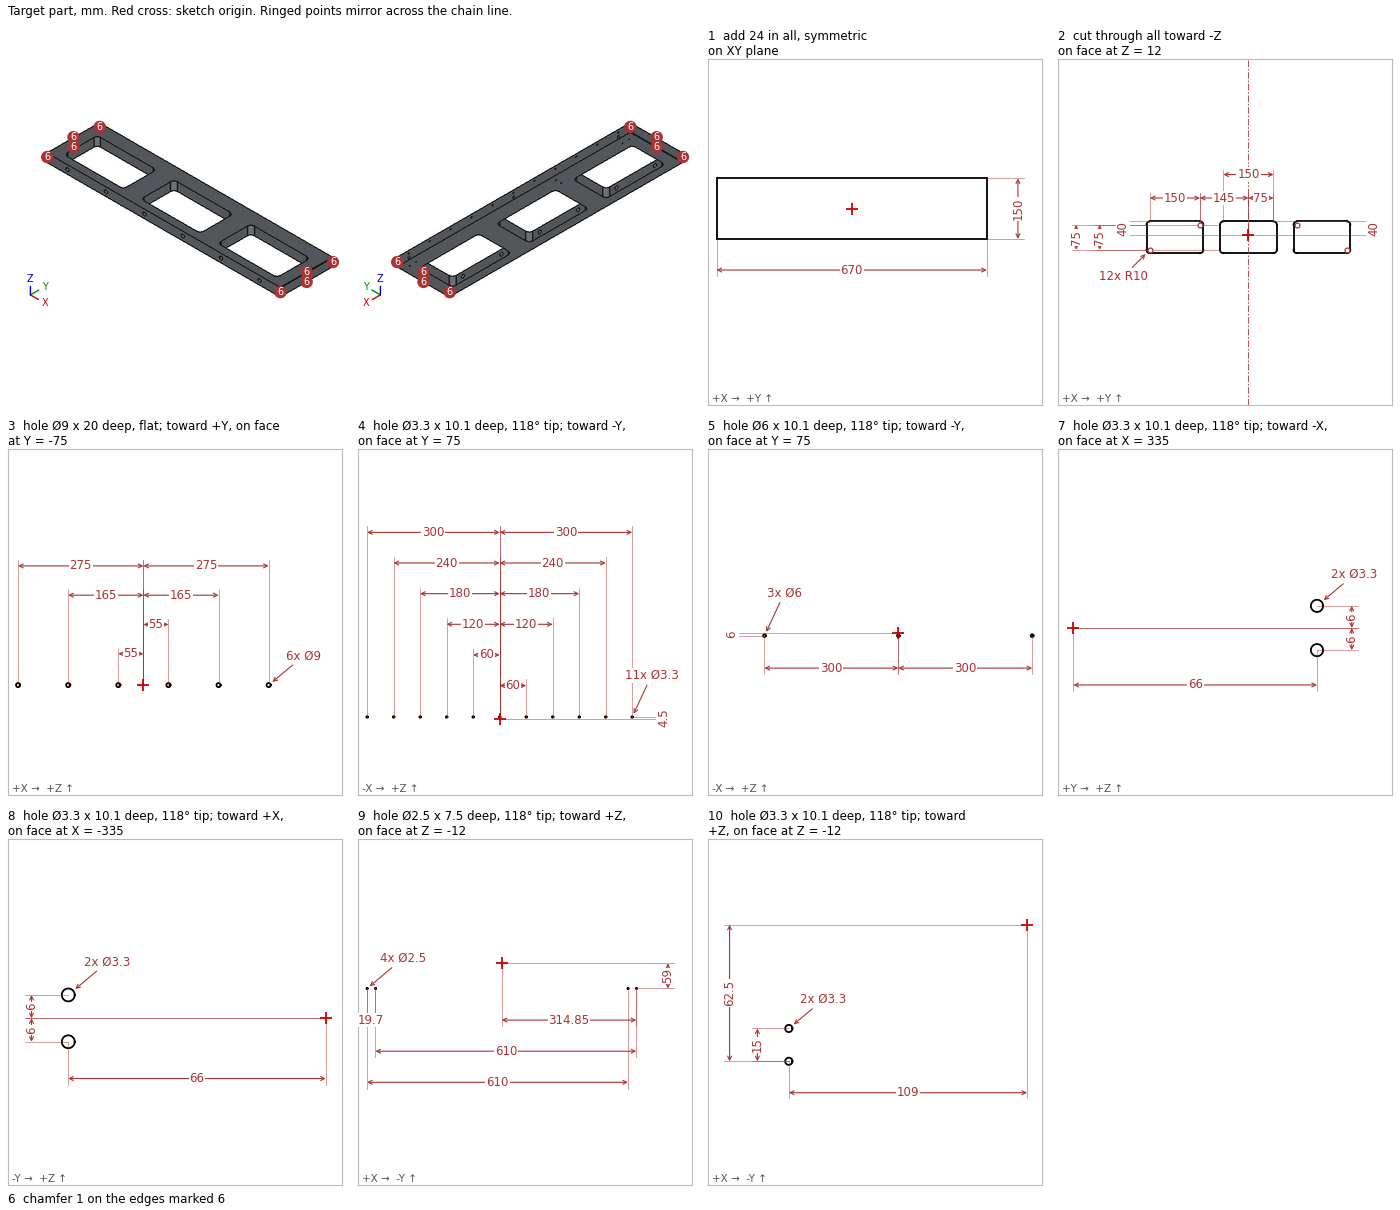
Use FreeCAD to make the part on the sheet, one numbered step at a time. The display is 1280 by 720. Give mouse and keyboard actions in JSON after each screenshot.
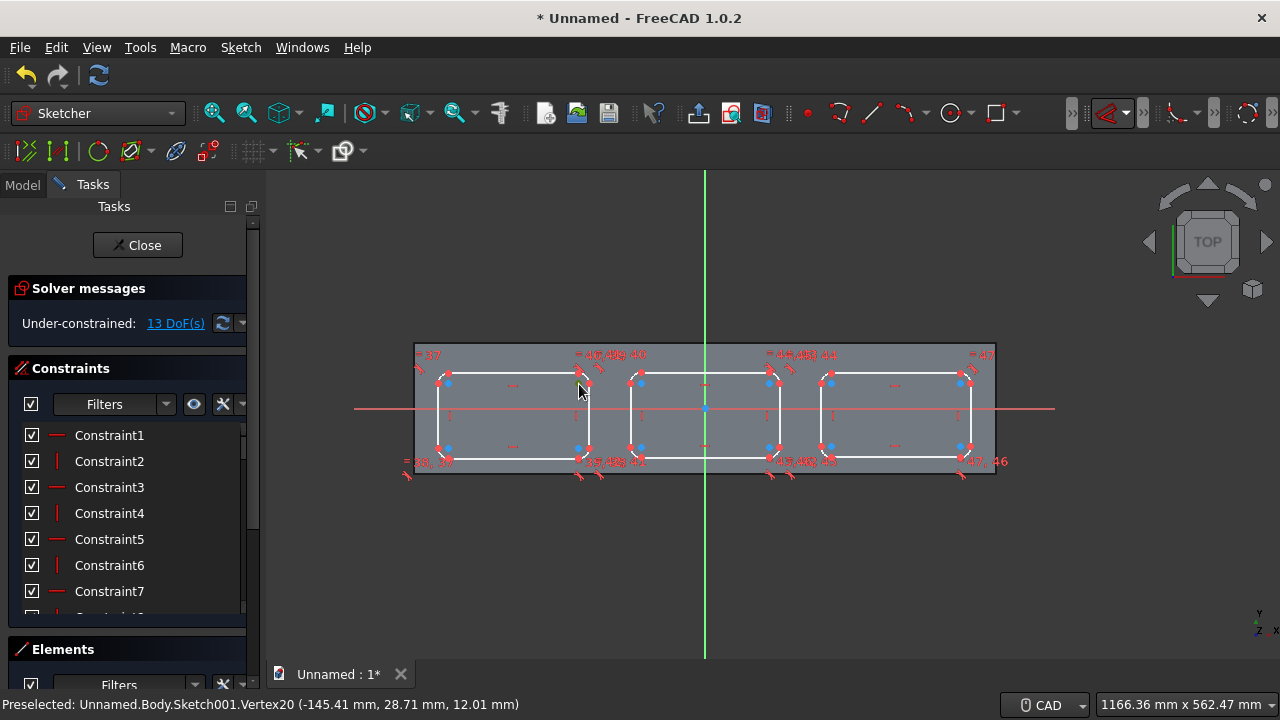
{"action": "left_click", "coordinate": [832, 384]}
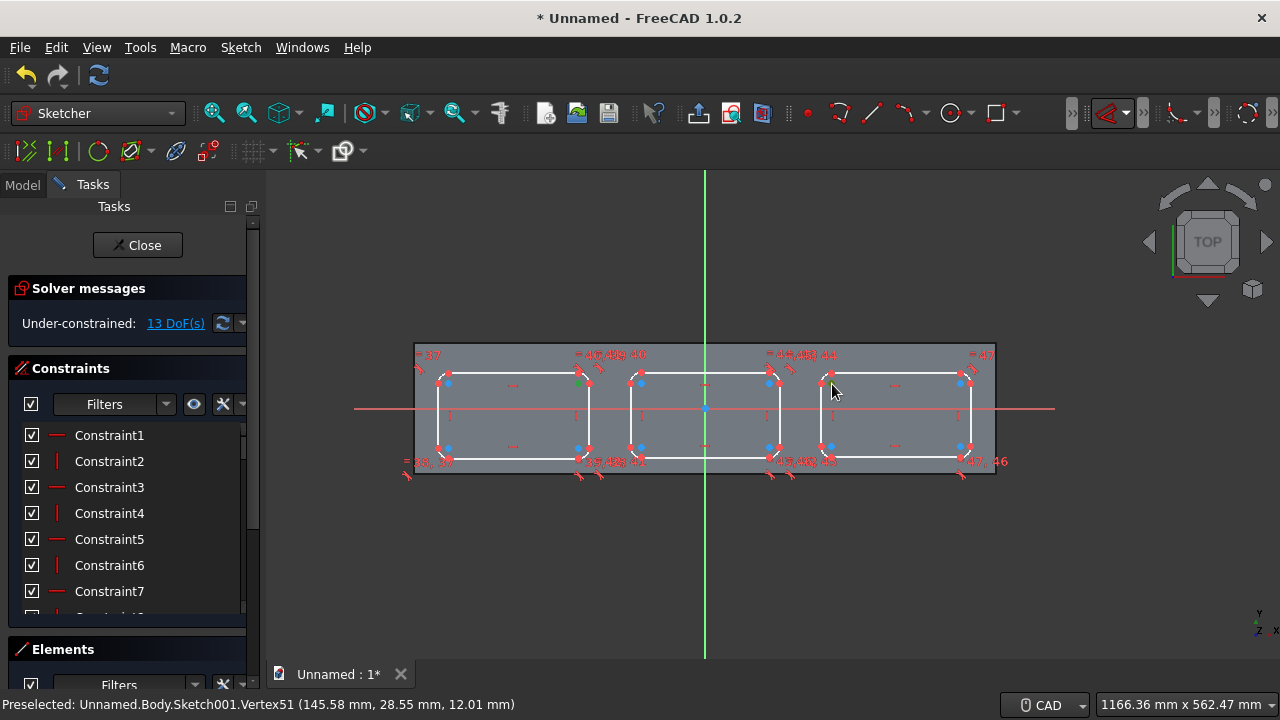
{"action": "left_click", "coordinate": [705, 600]}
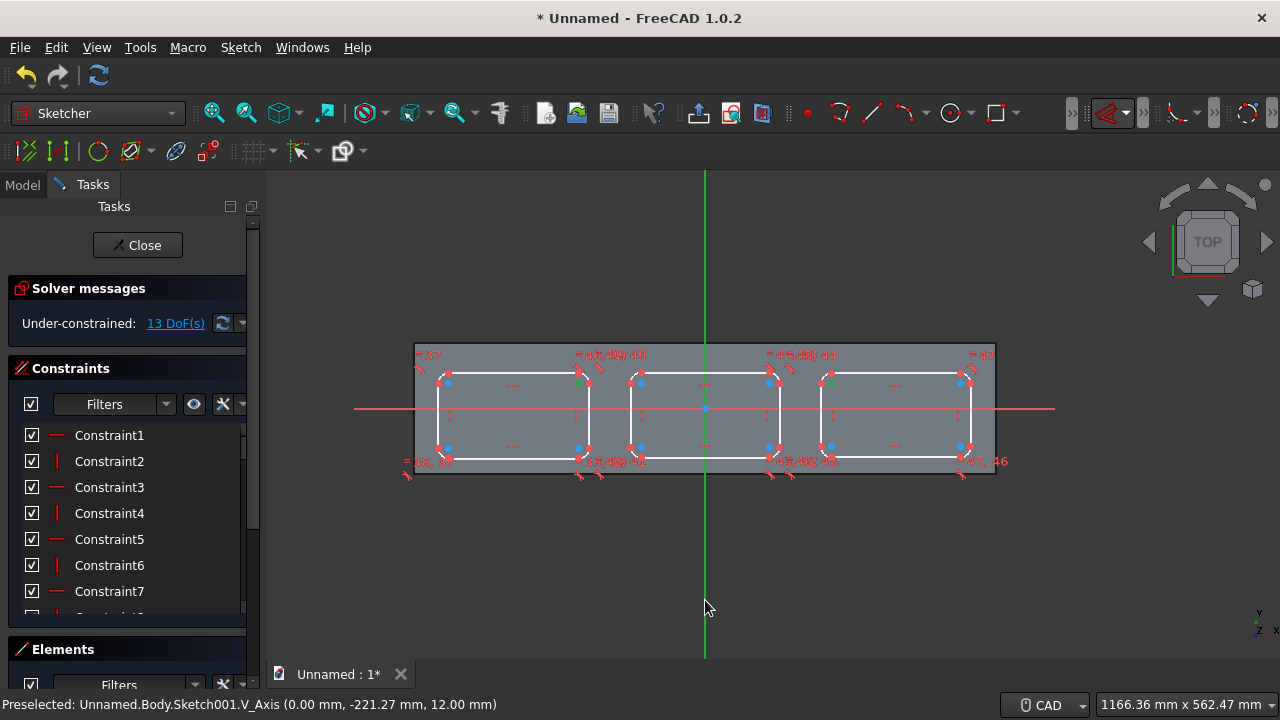
{"action": "key", "text": "s"}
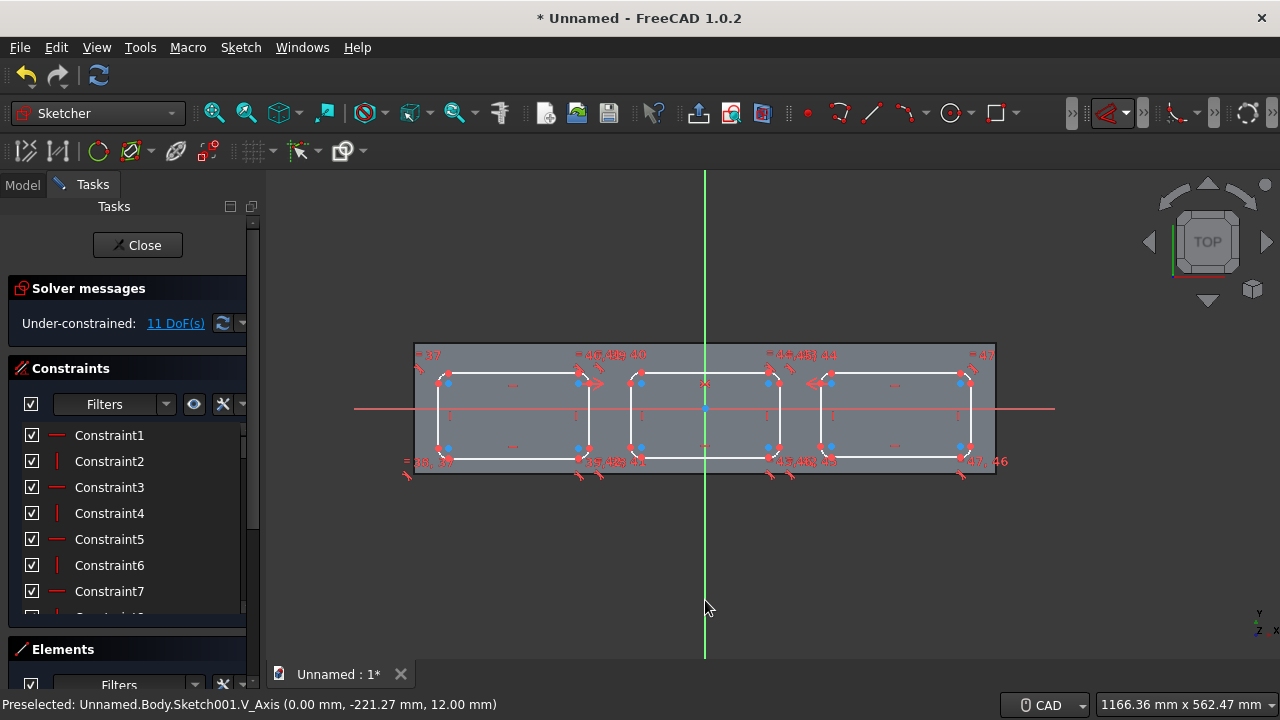
{"action": "left_click", "coordinate": [449, 448]}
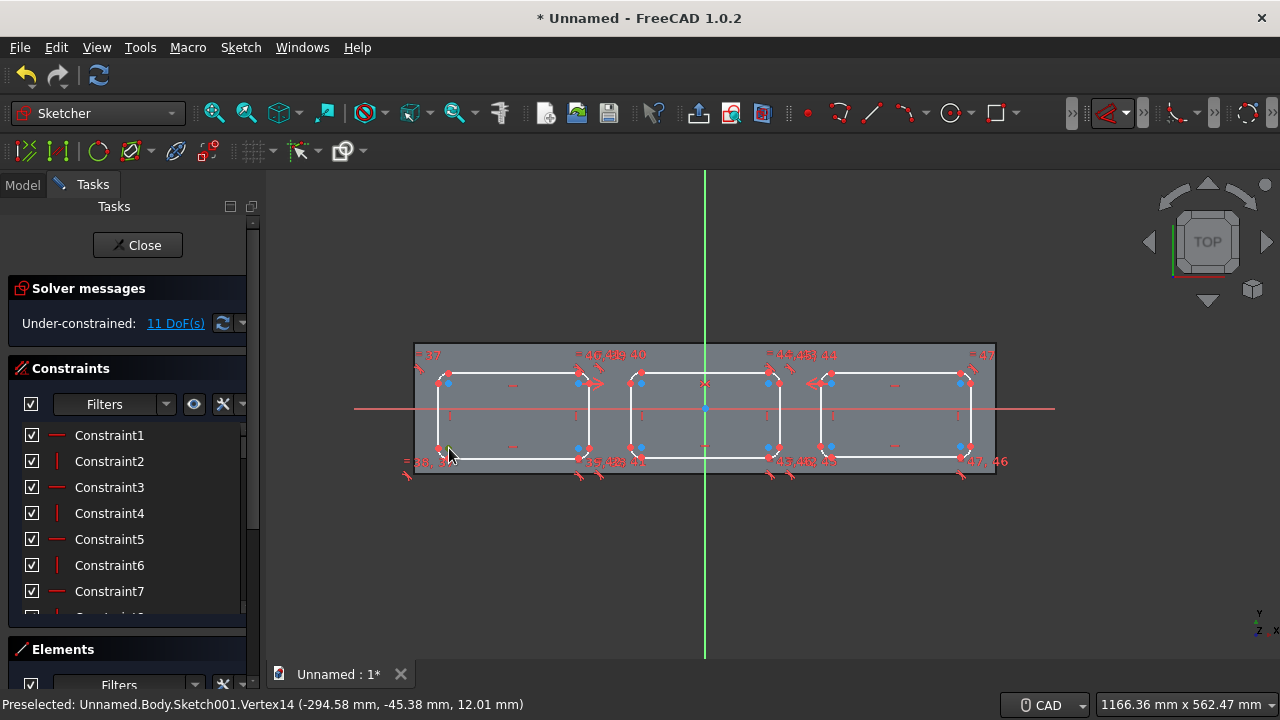
{"action": "left_click", "coordinate": [960, 447]}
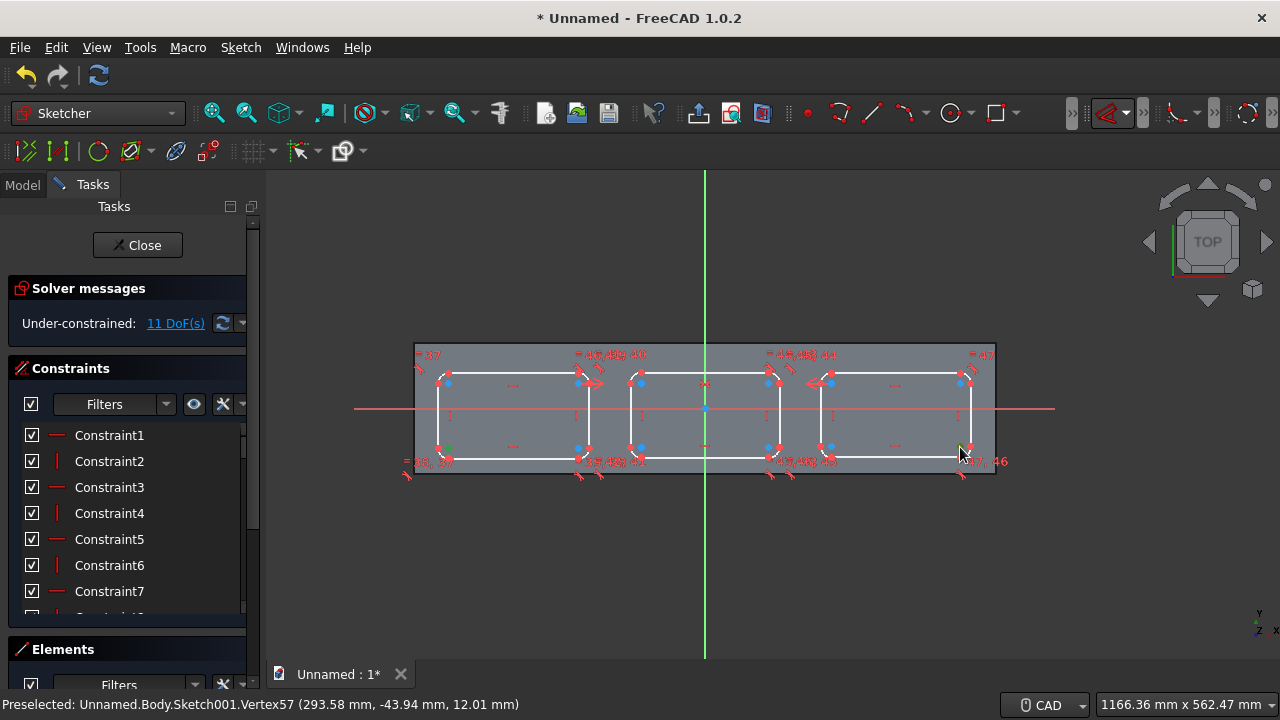
{"action": "left_click", "coordinate": [705, 600]}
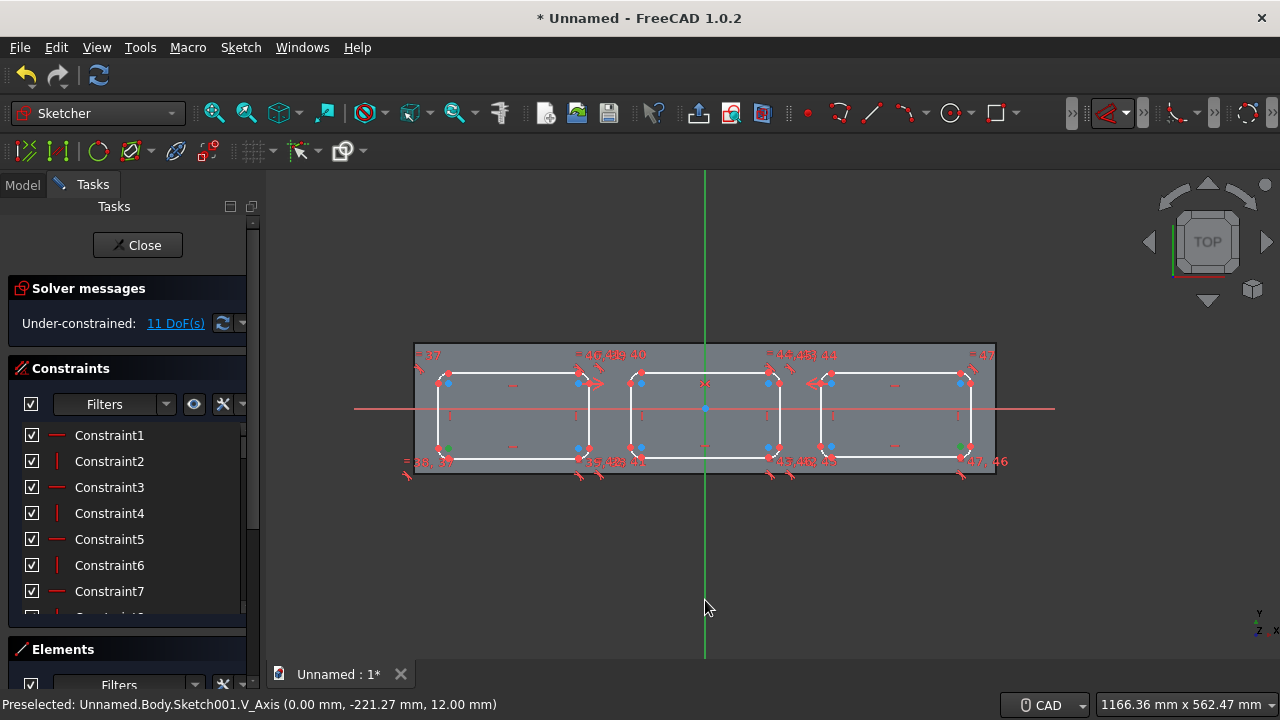
{"action": "key", "text": "s"}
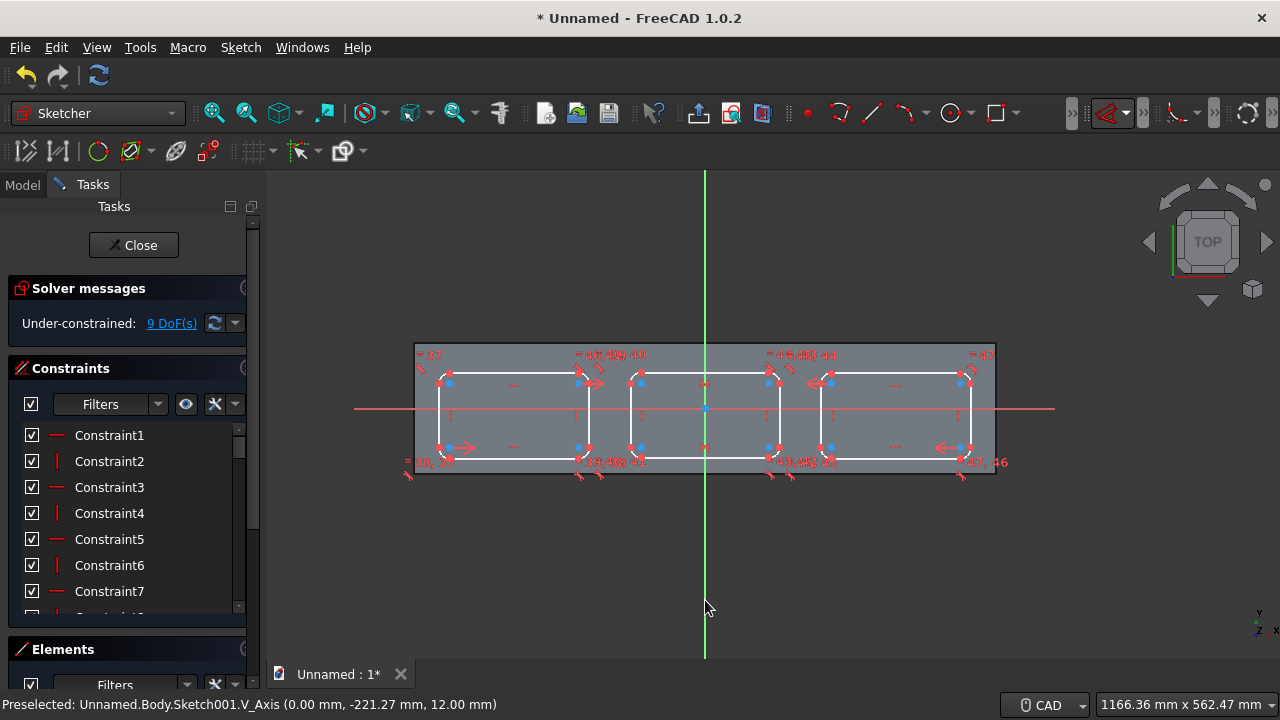
{"action": "left_click", "coordinate": [1106, 114]}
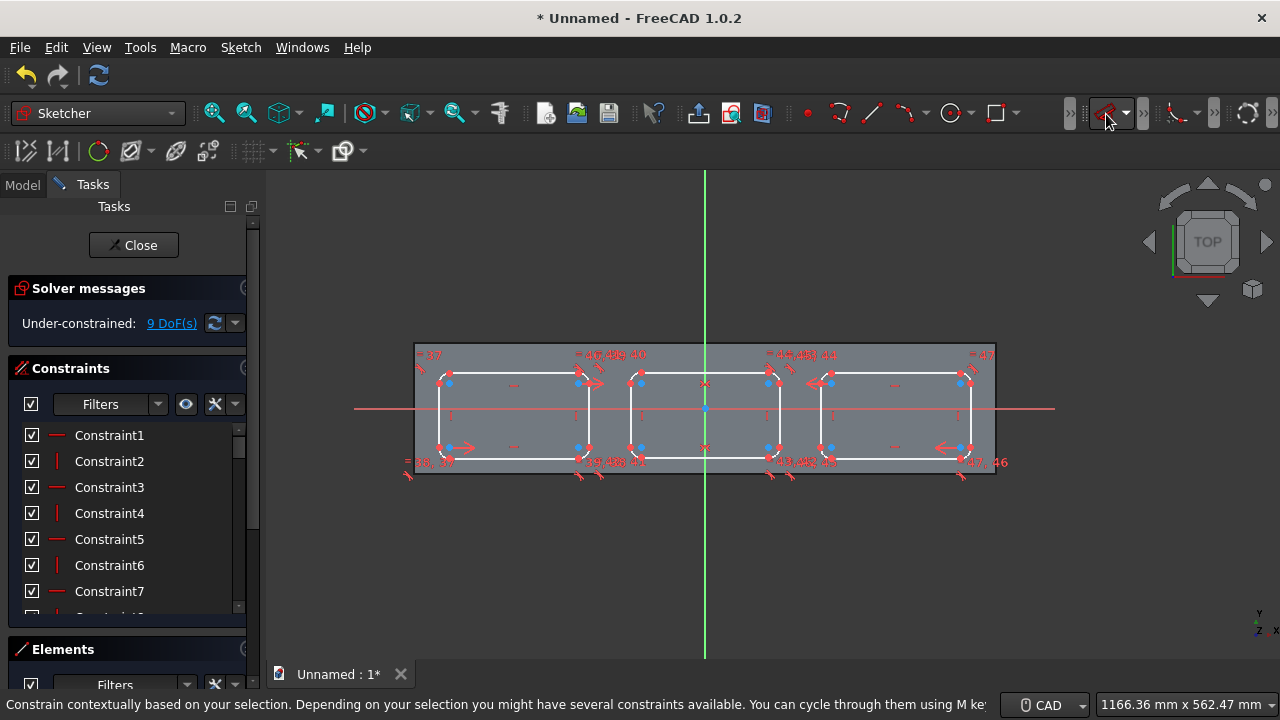
{"action": "scroll", "coordinate": [442, 376], "scroll_direction": "up", "scroll_amount": 8}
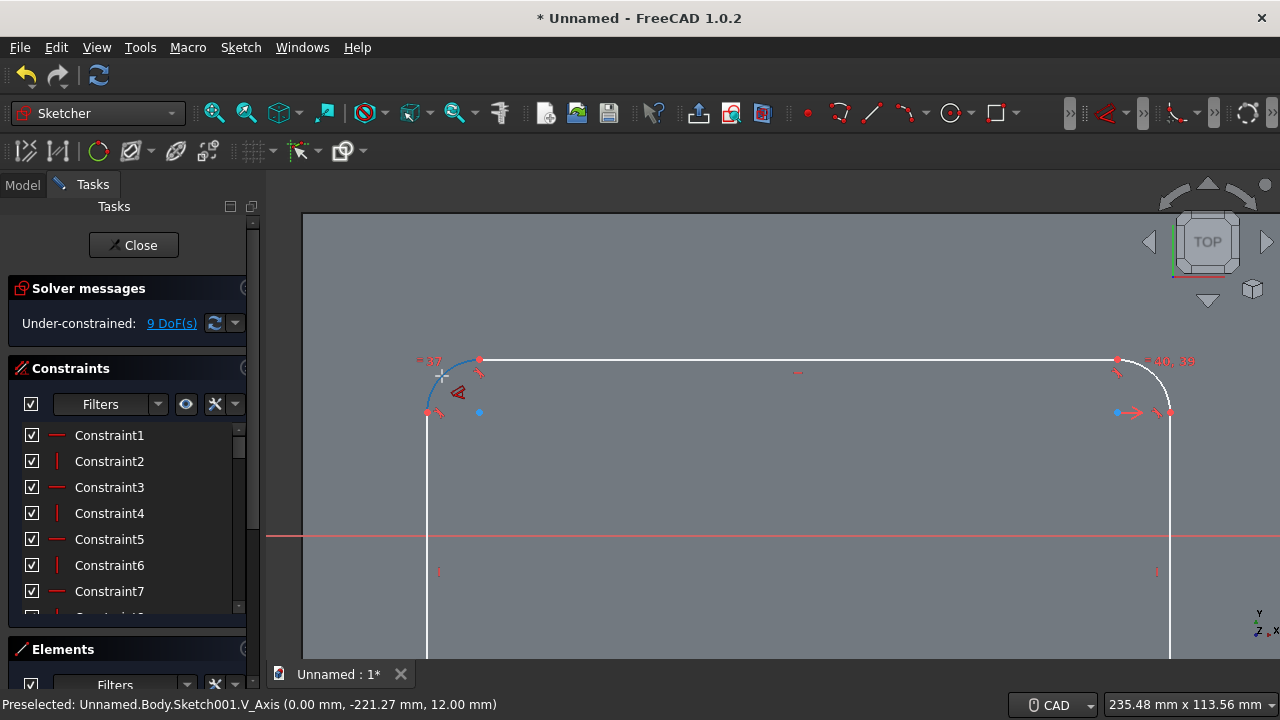
{"action": "left_click", "coordinate": [443, 375]}
{"action": "left_click", "coordinate": [421, 352]}